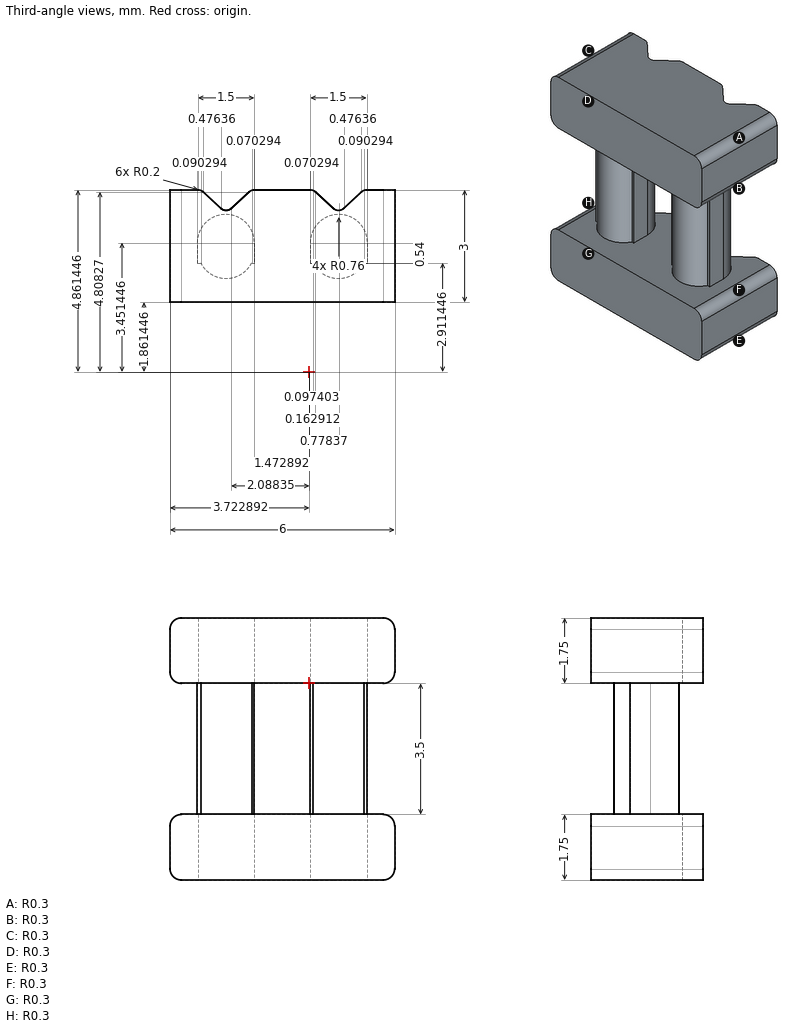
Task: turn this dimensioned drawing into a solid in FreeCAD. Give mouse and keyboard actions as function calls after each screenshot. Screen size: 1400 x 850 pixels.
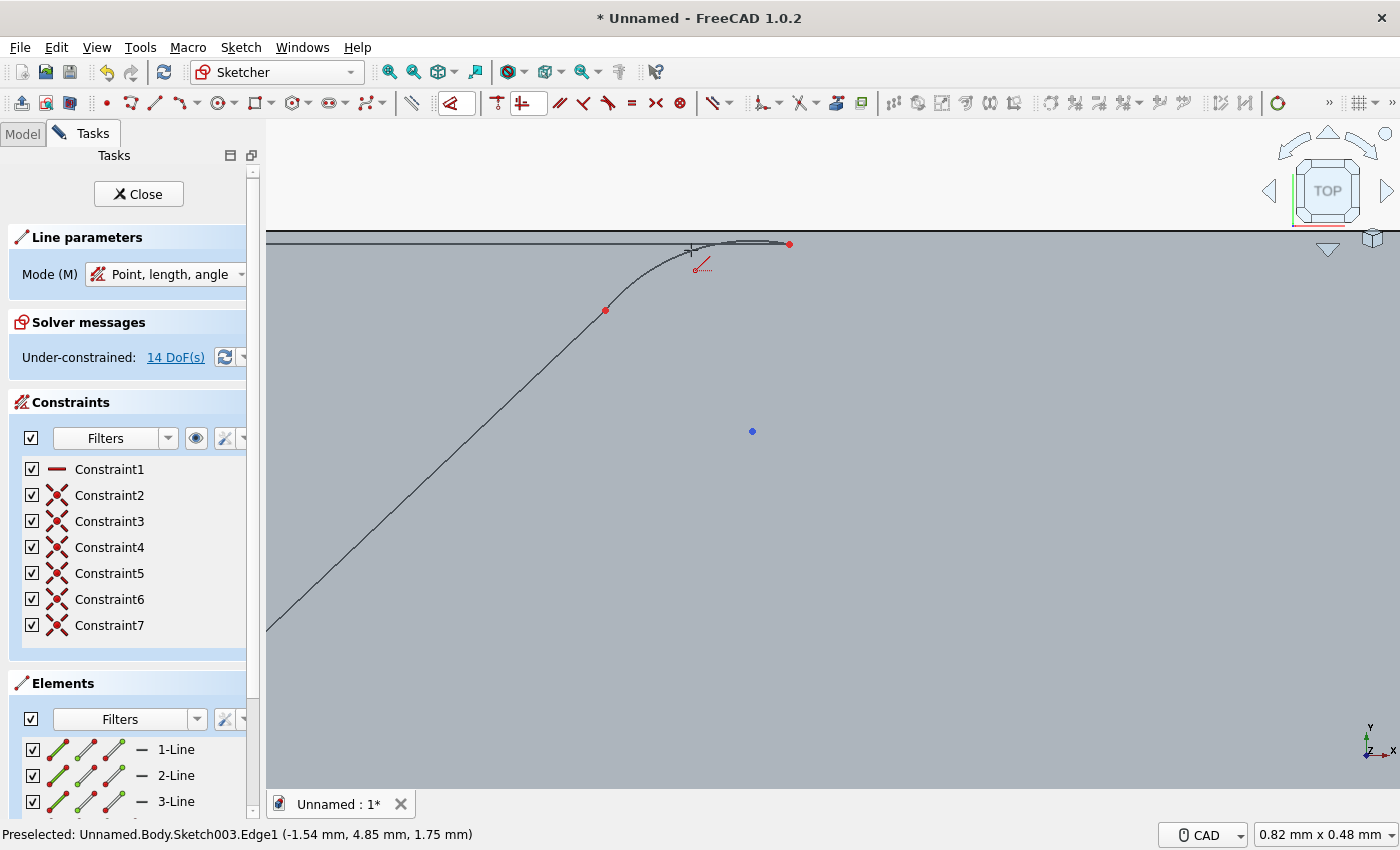
scroll(695, 250, down, 14)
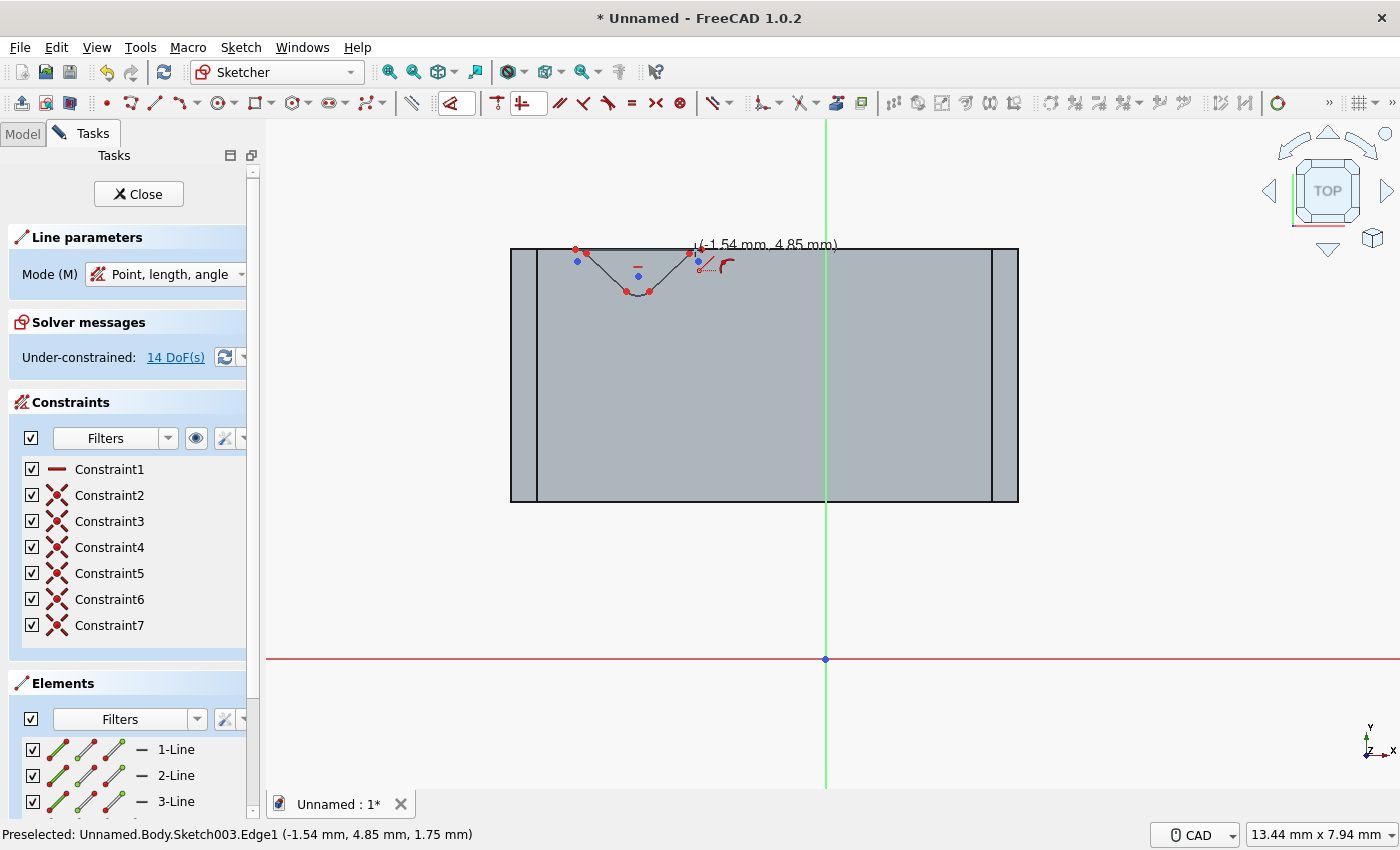
click(839, 254)
click(880, 291)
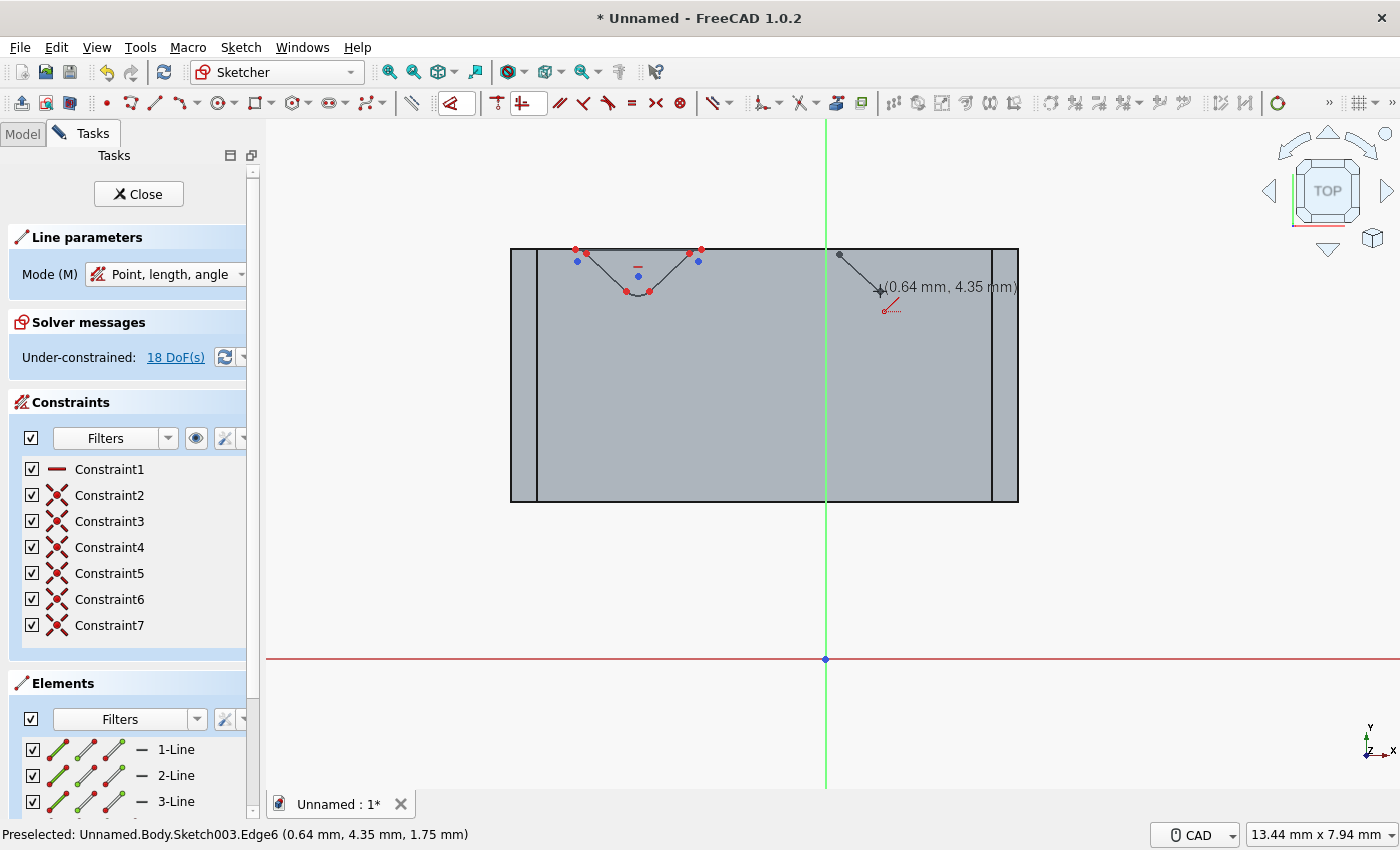
click(903, 291)
click(943, 254)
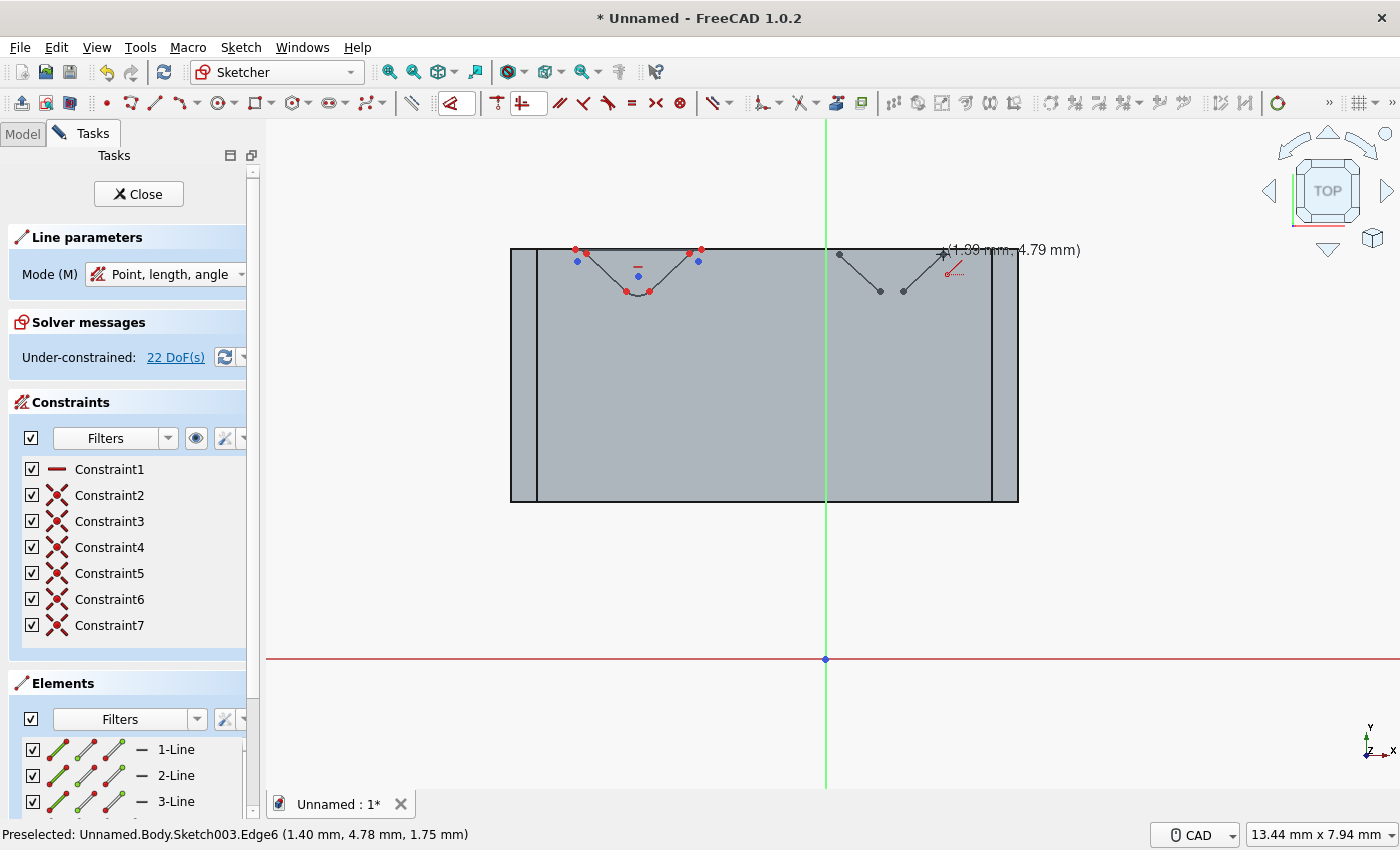
scroll(954, 249, up, 2)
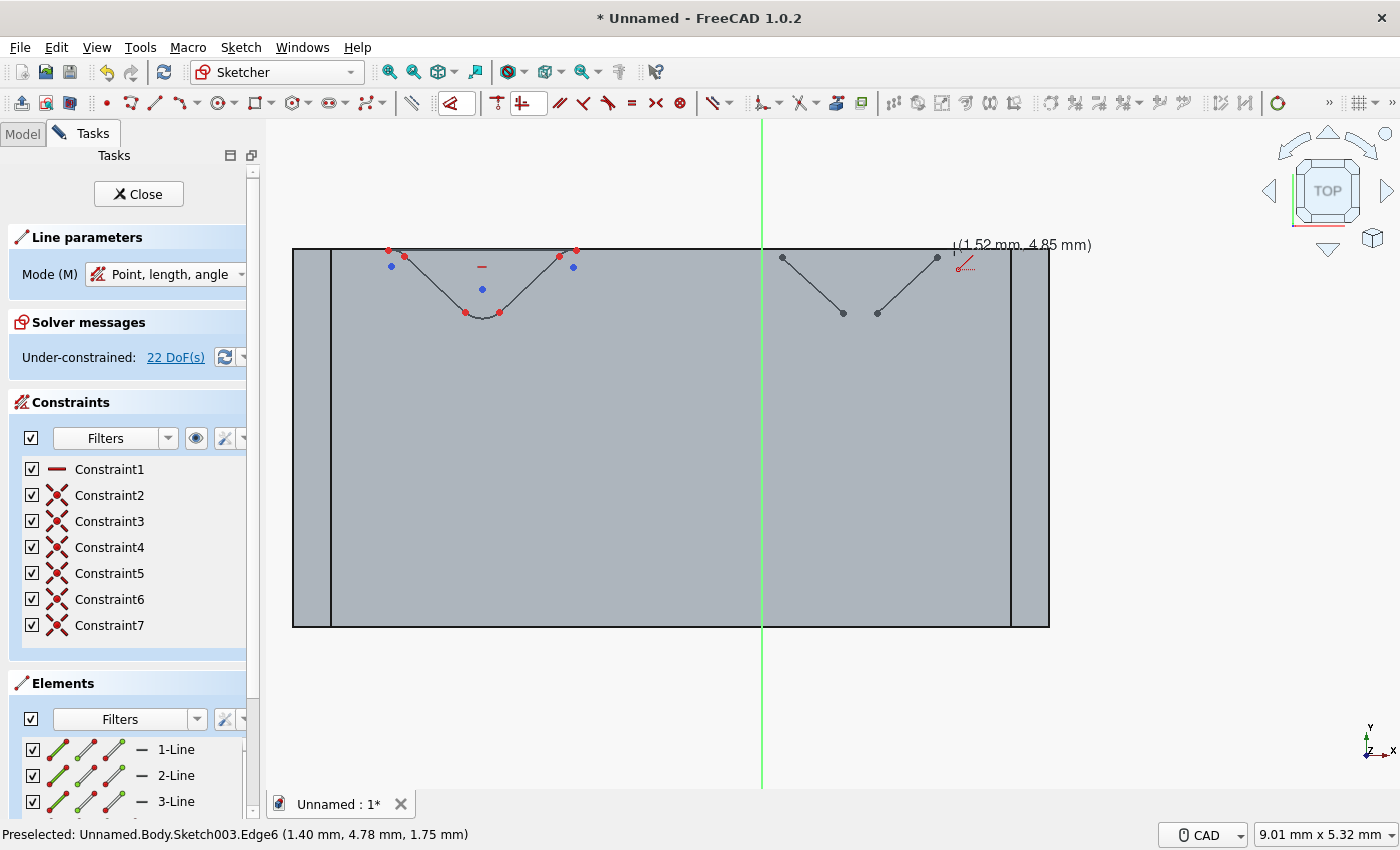
click(954, 249)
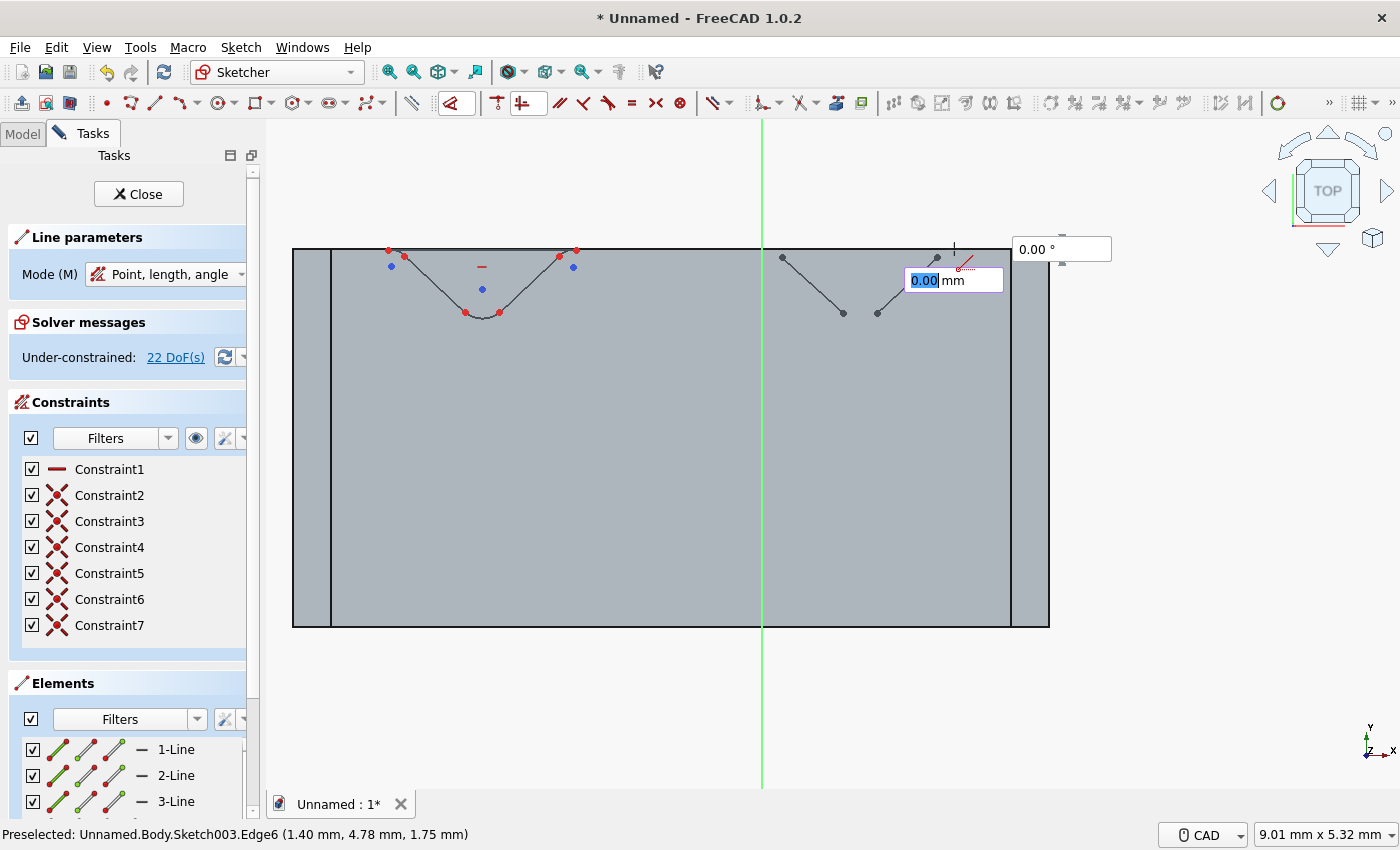
scroll(766, 249, up, 8)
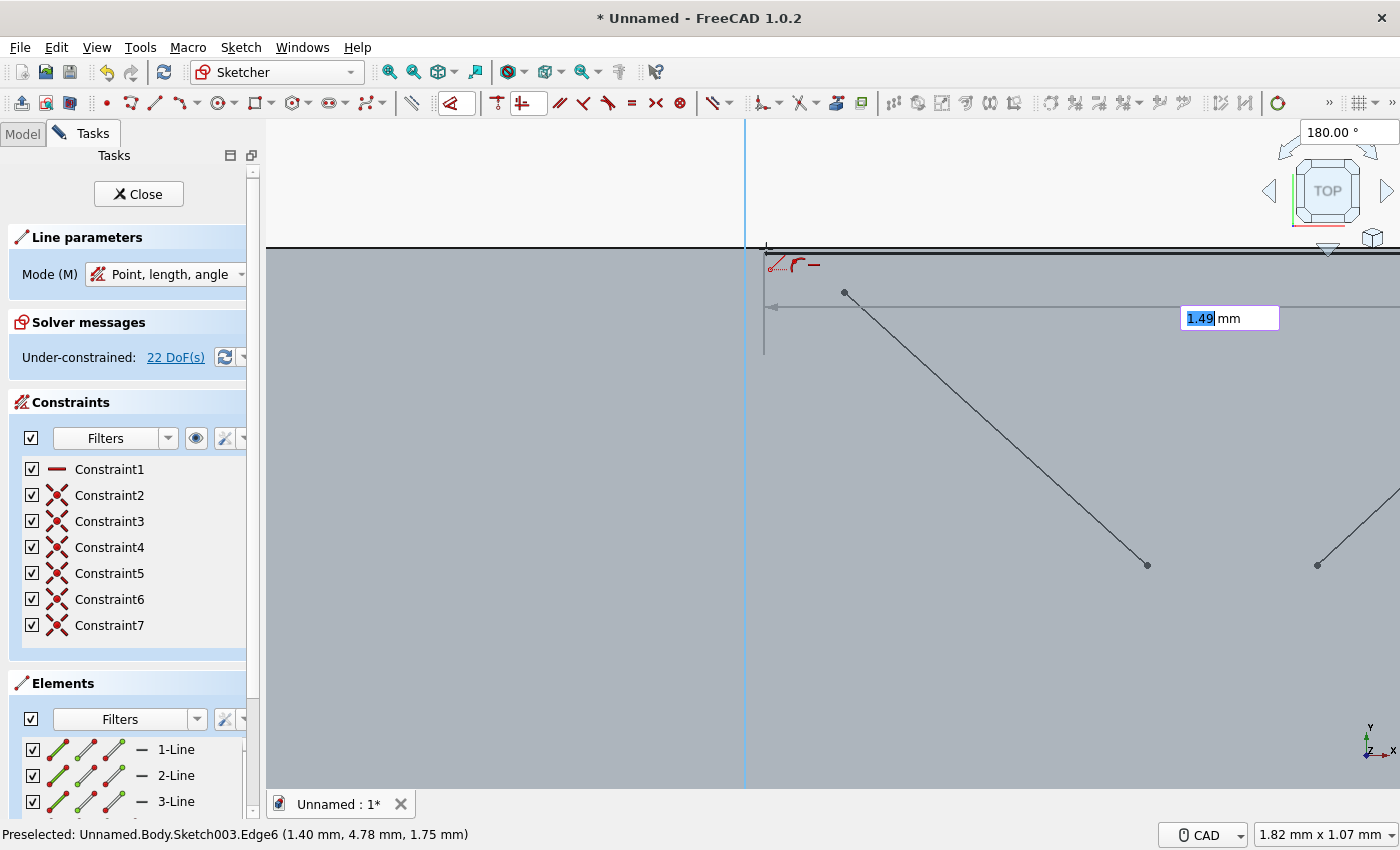
click(762, 248)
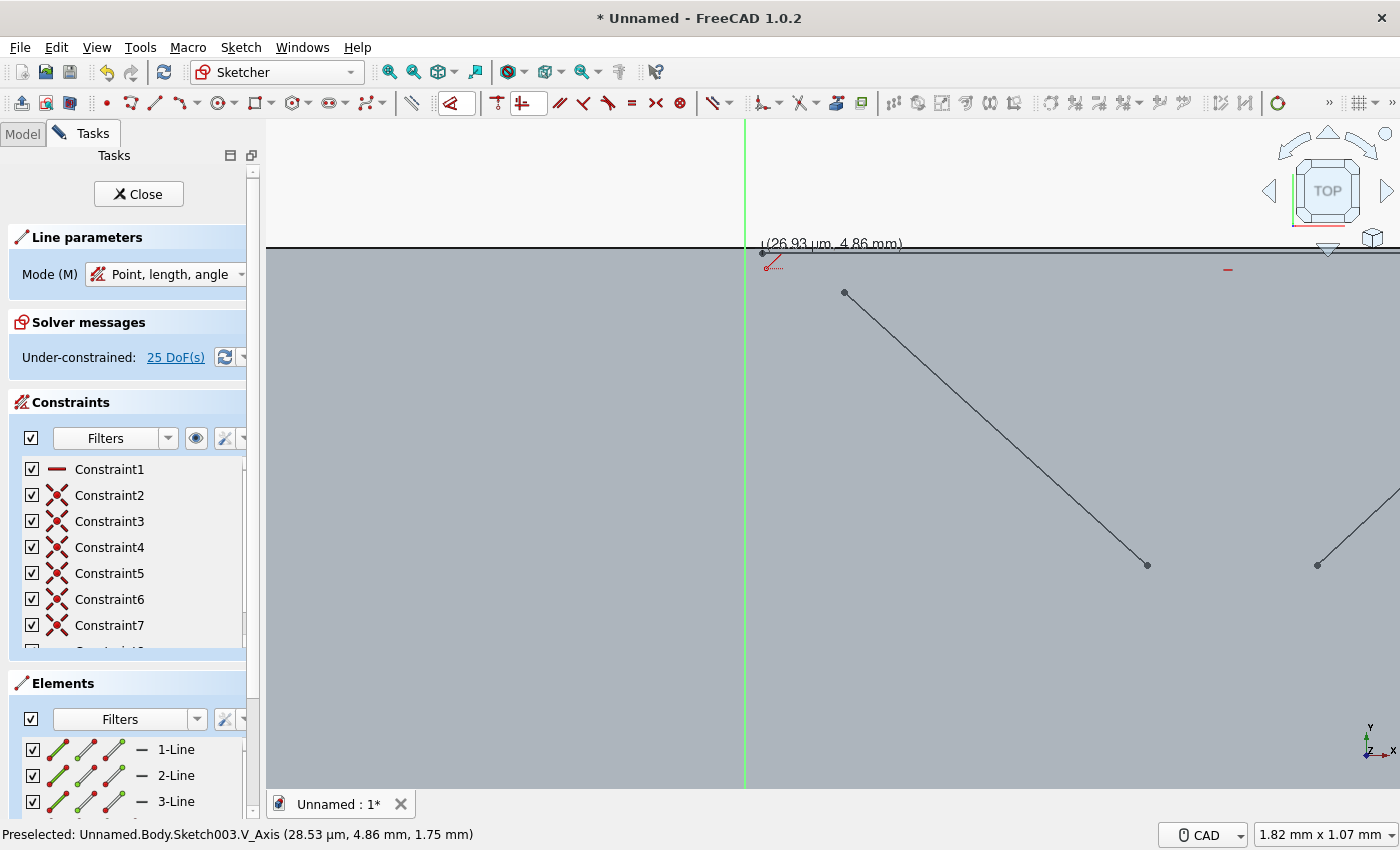
click(180, 104)